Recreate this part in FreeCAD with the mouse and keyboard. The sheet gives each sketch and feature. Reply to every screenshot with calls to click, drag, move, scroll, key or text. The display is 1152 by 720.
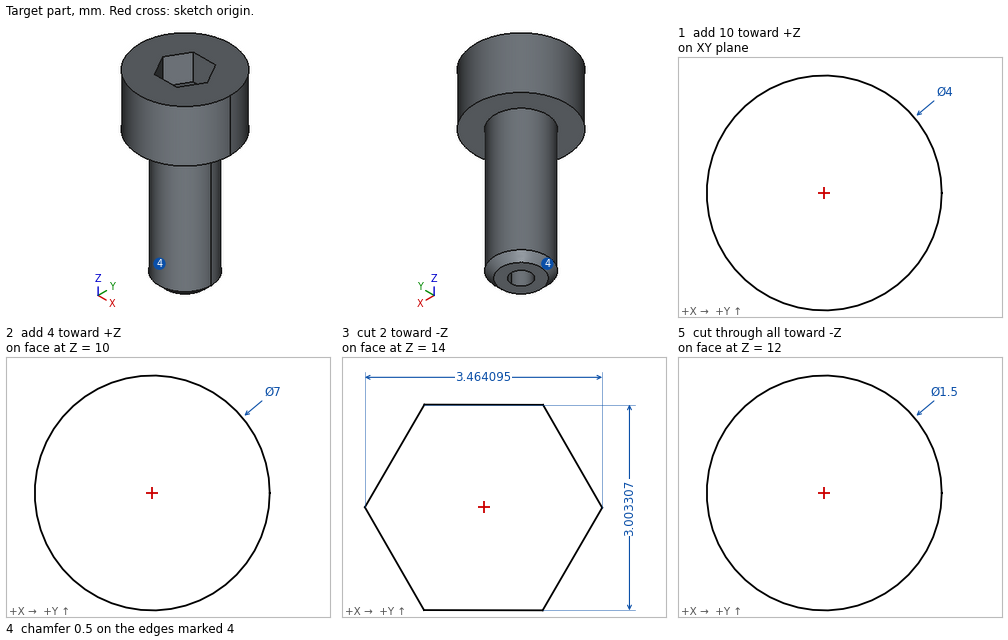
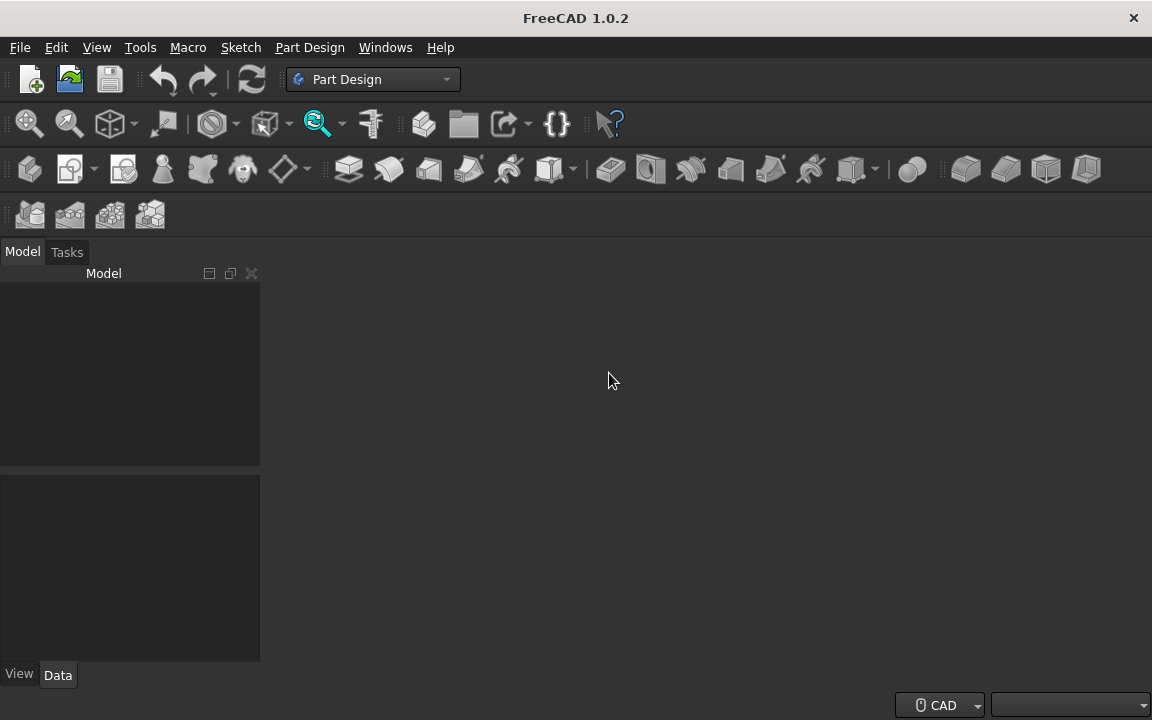
key(ctrl+n)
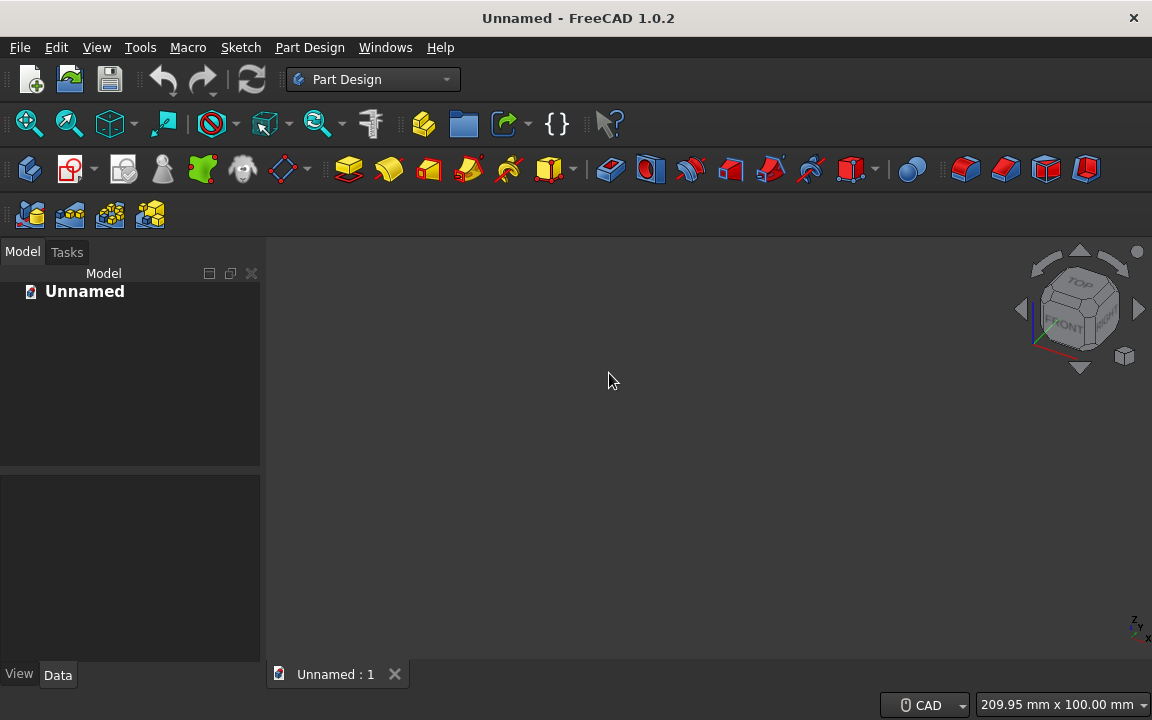
click(70, 170)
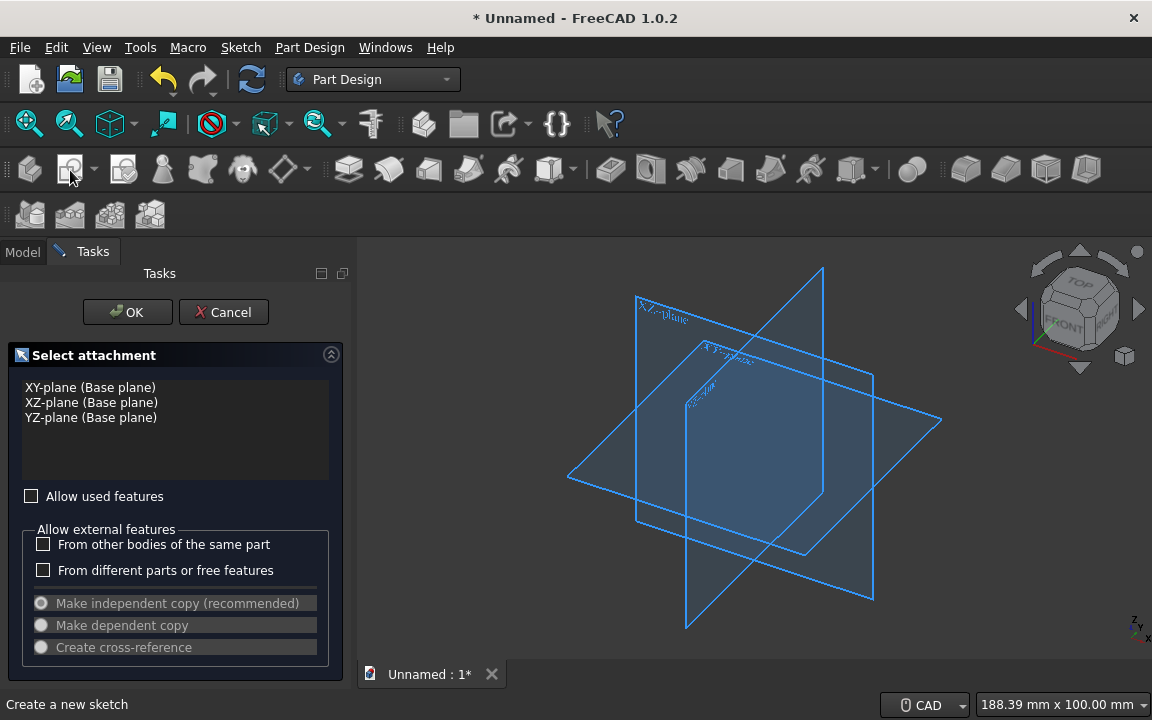
click(82, 388)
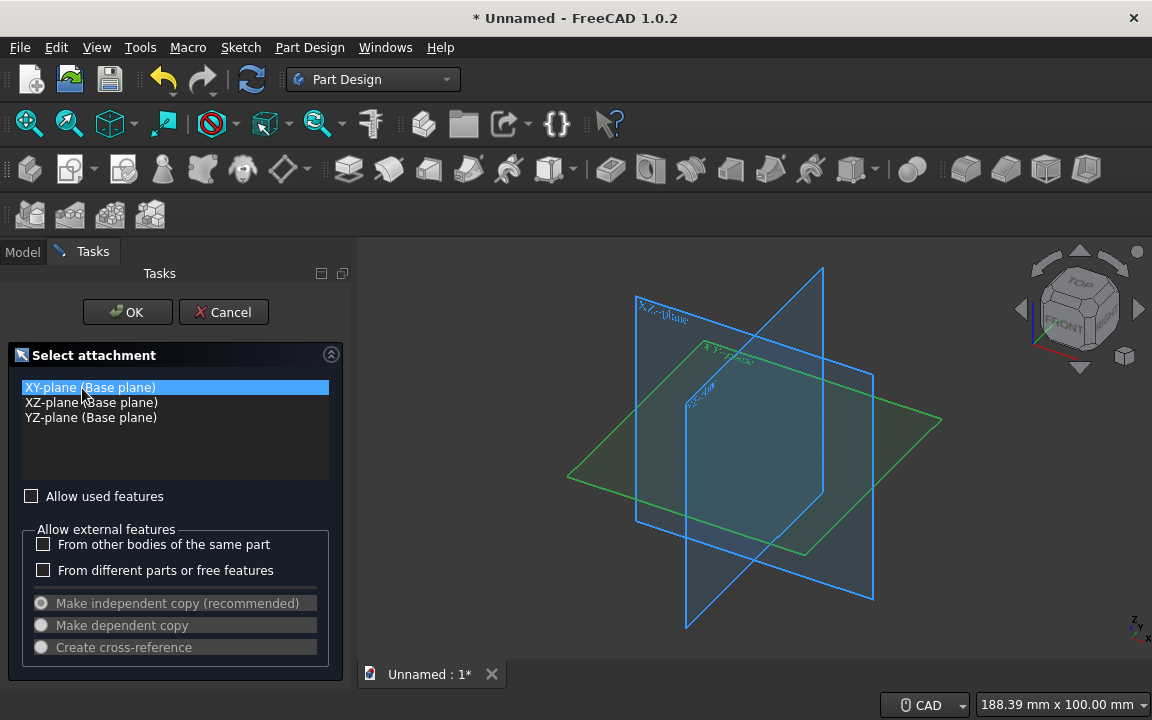
click(128, 312)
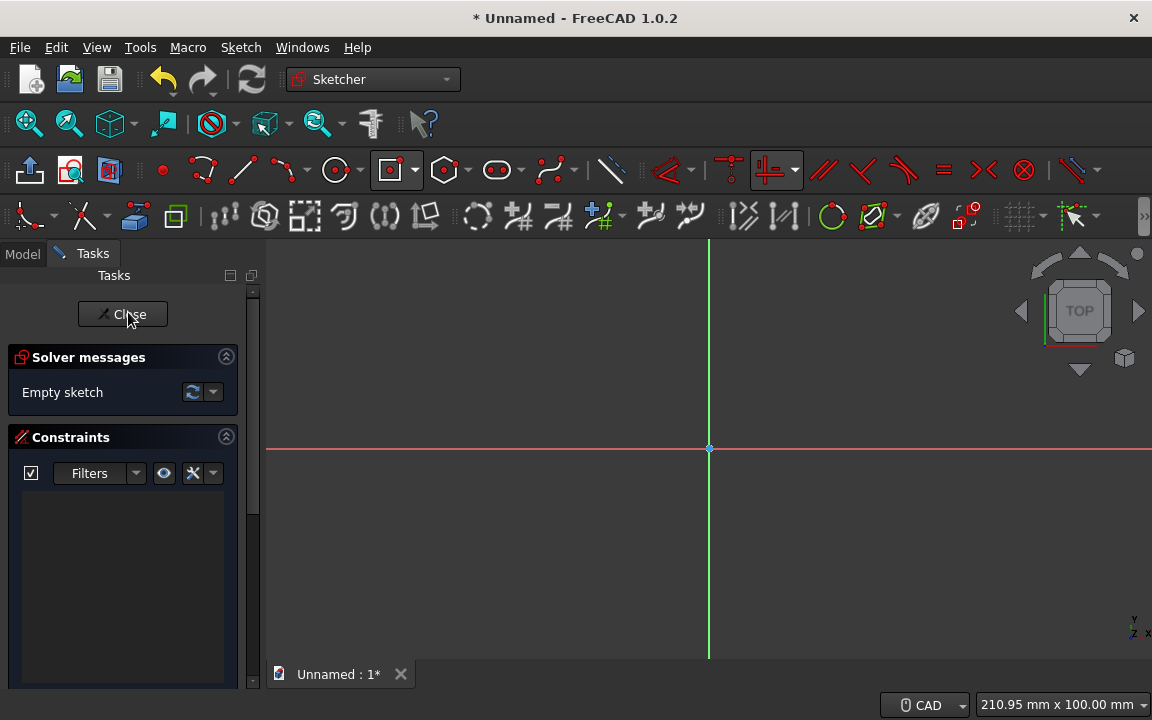
scroll(713, 449, up, 14)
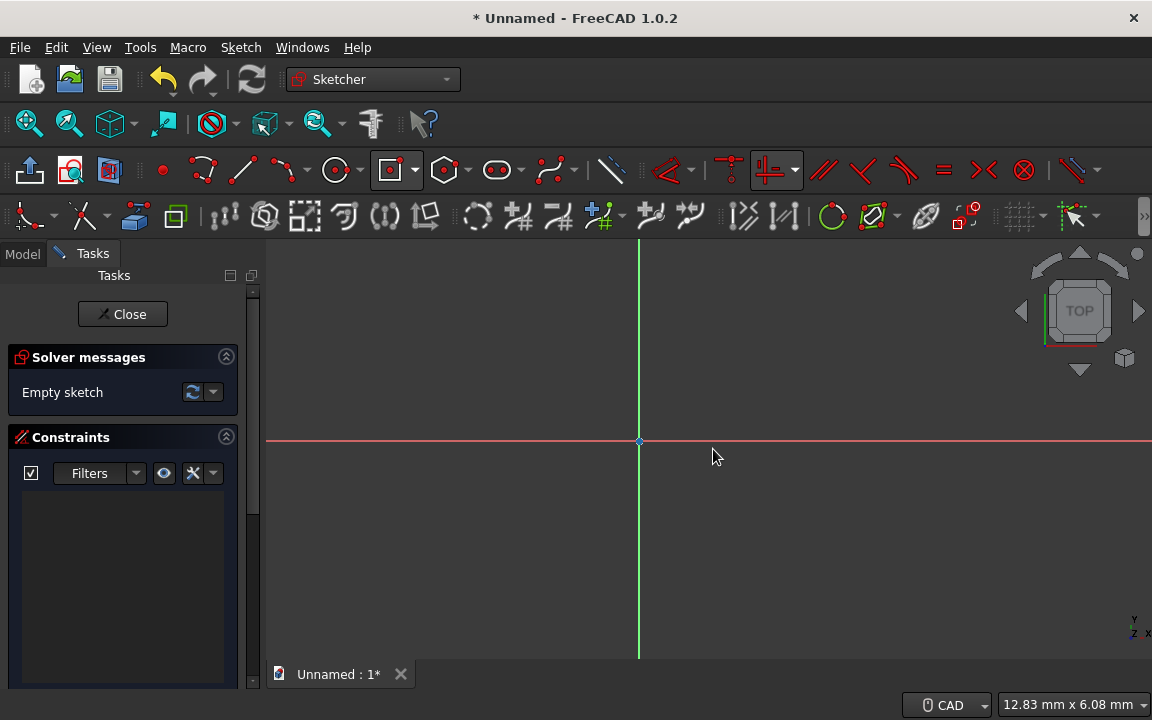
click(336, 170)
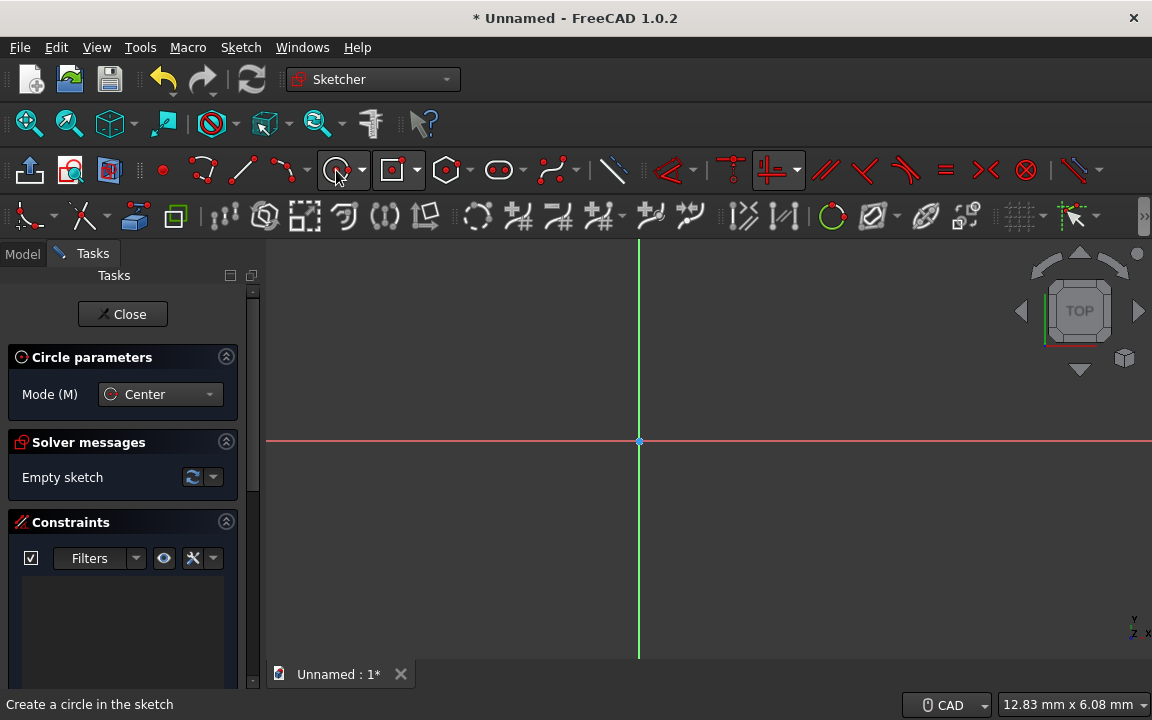
click(639, 441)
move(737, 344)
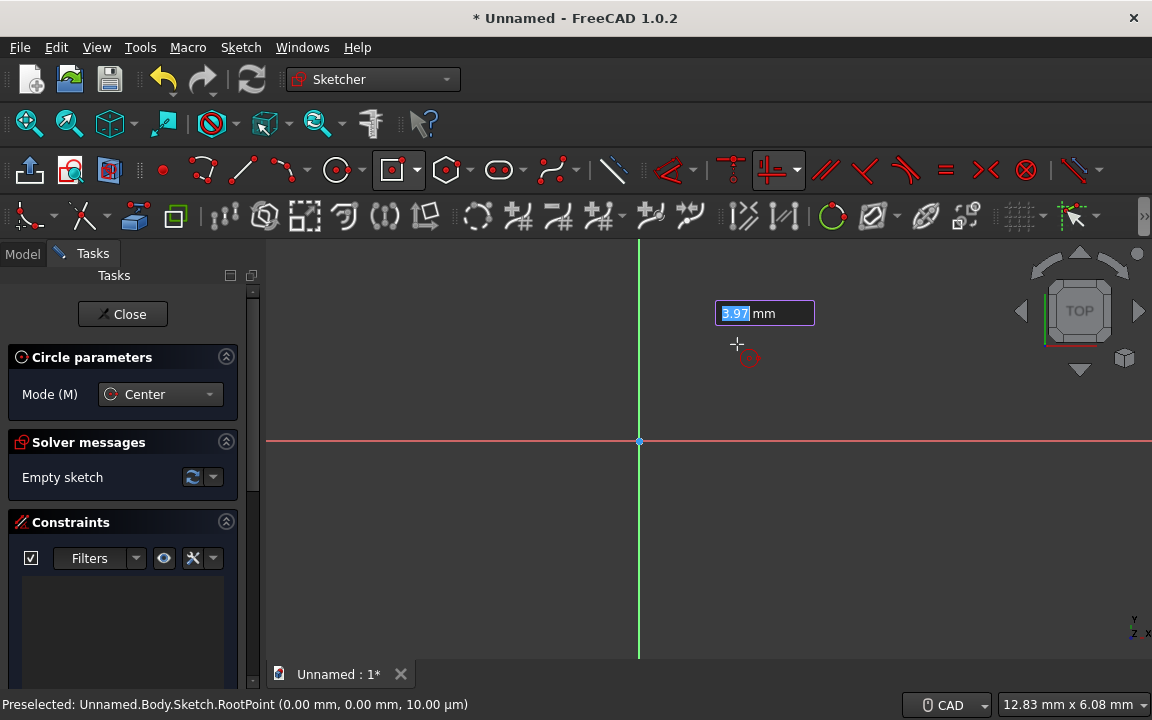
text(4)
key(Return)
key(Escape)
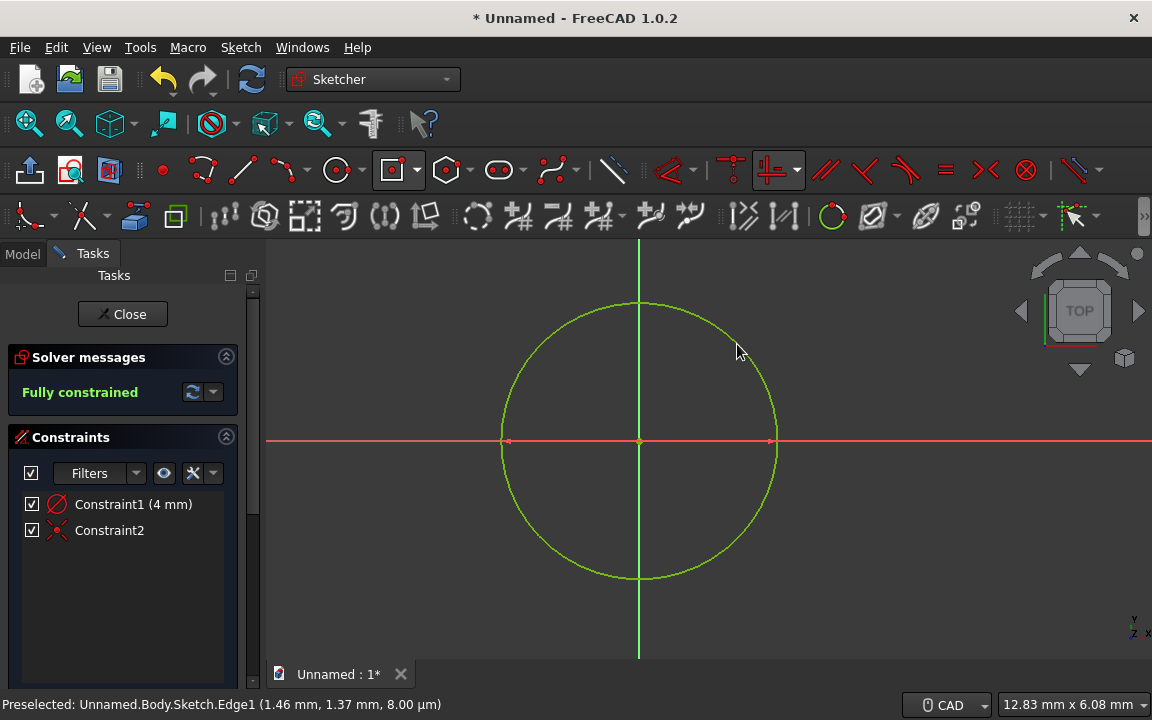
click(123, 314)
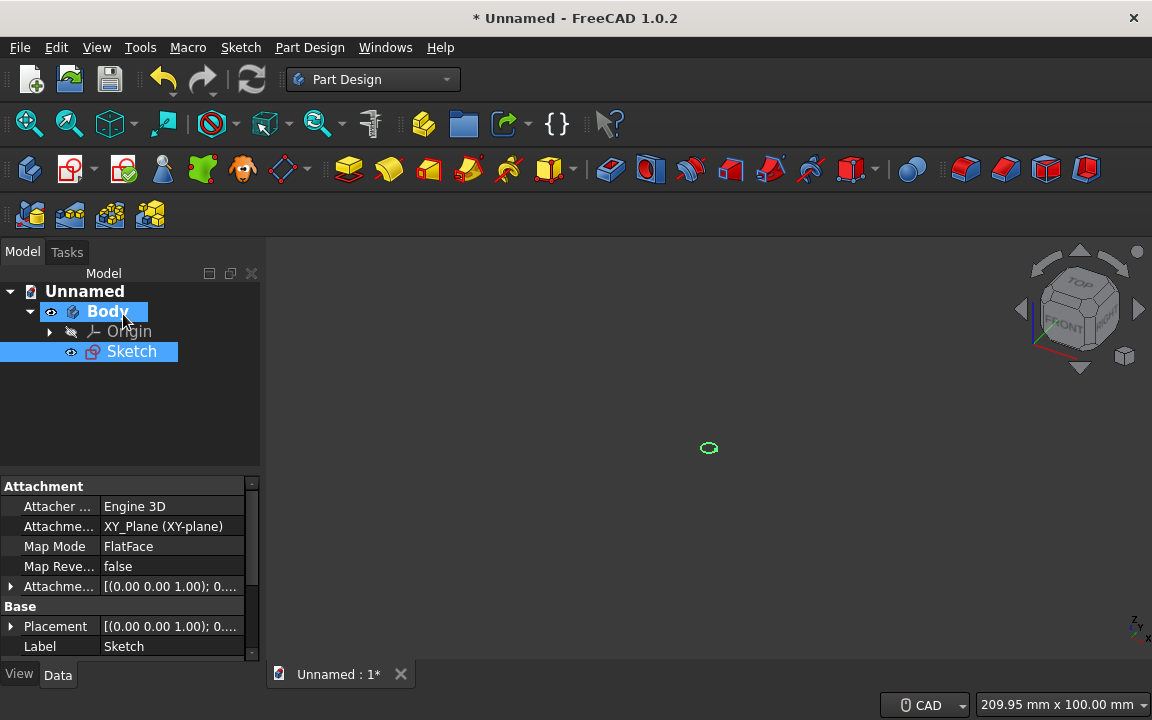
click(350, 170)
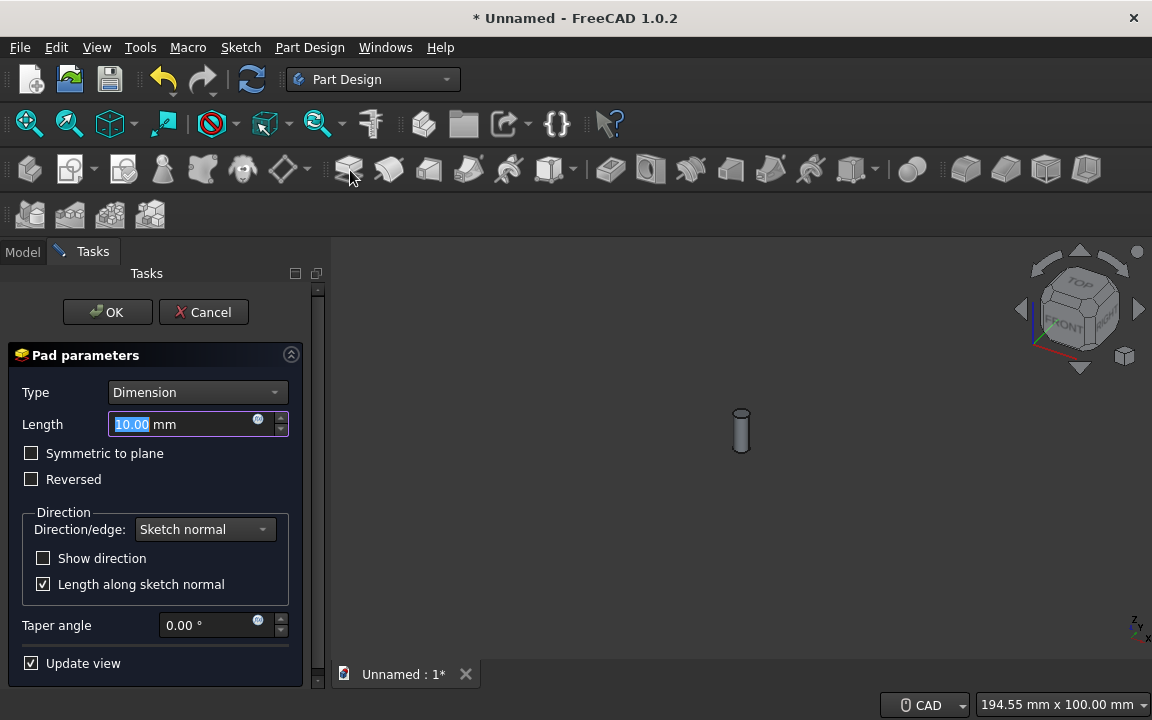
text(10)
key(Tab)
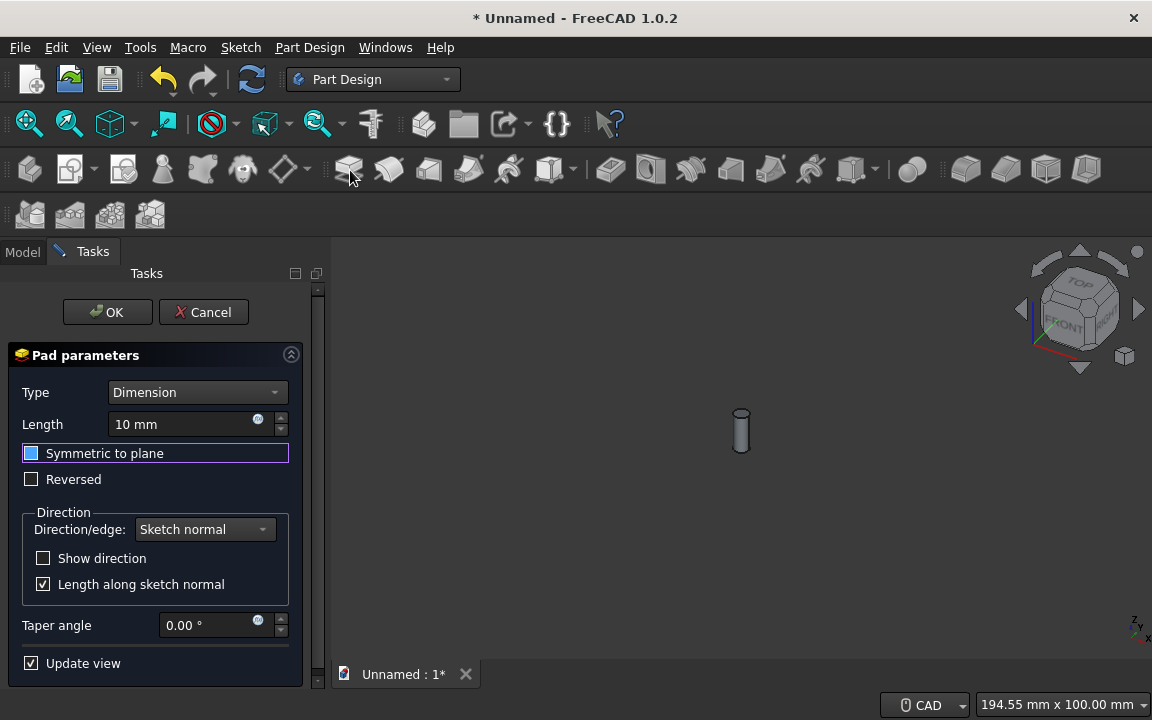
click(108, 312)